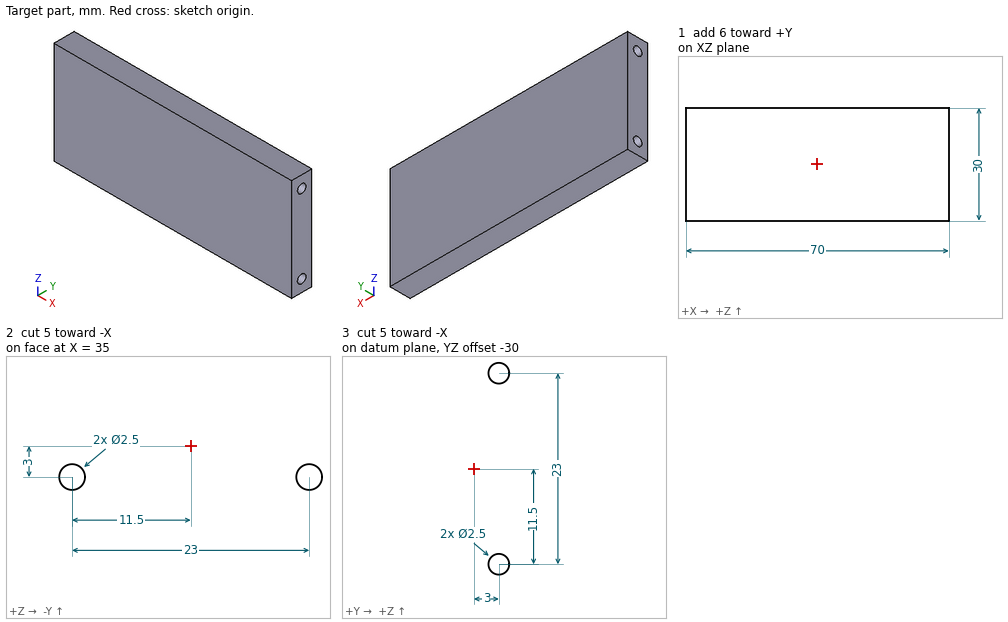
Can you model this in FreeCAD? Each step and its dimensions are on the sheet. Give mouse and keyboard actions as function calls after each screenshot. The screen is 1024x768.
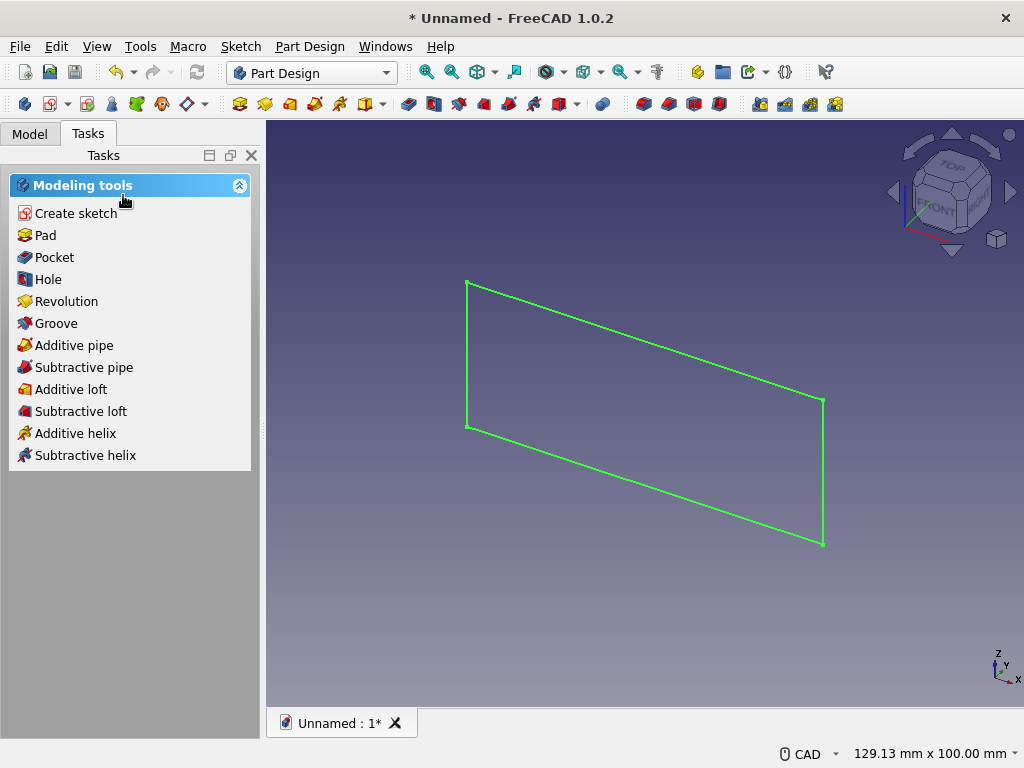
click(240, 104)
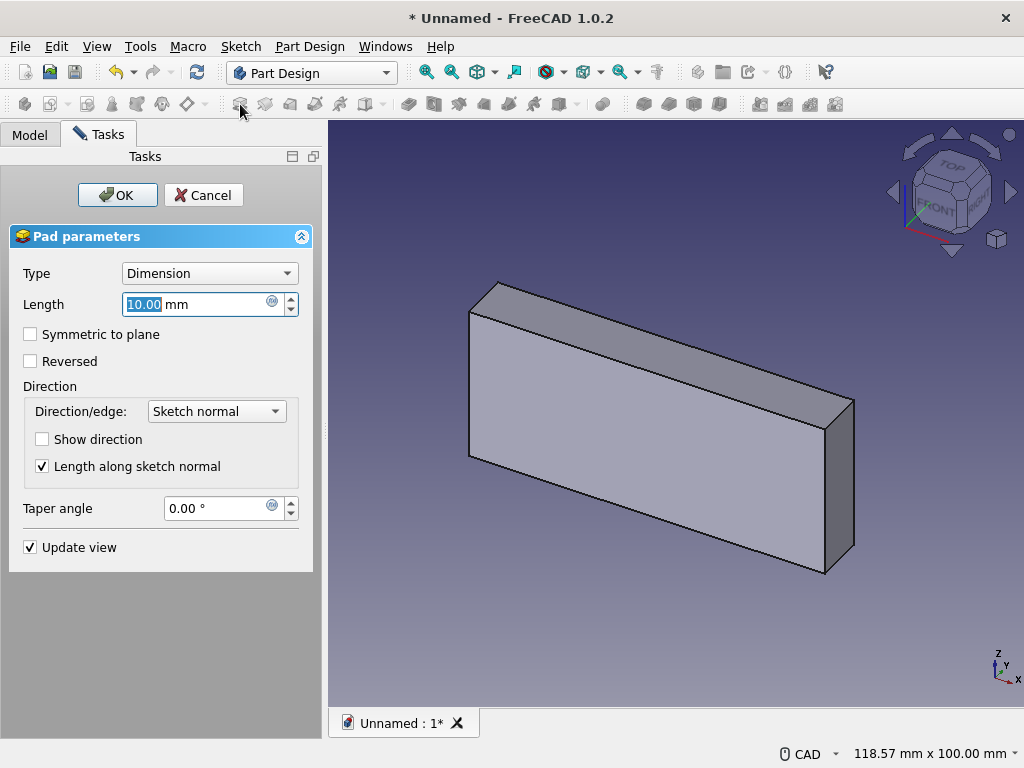
text(6)
key(Tab)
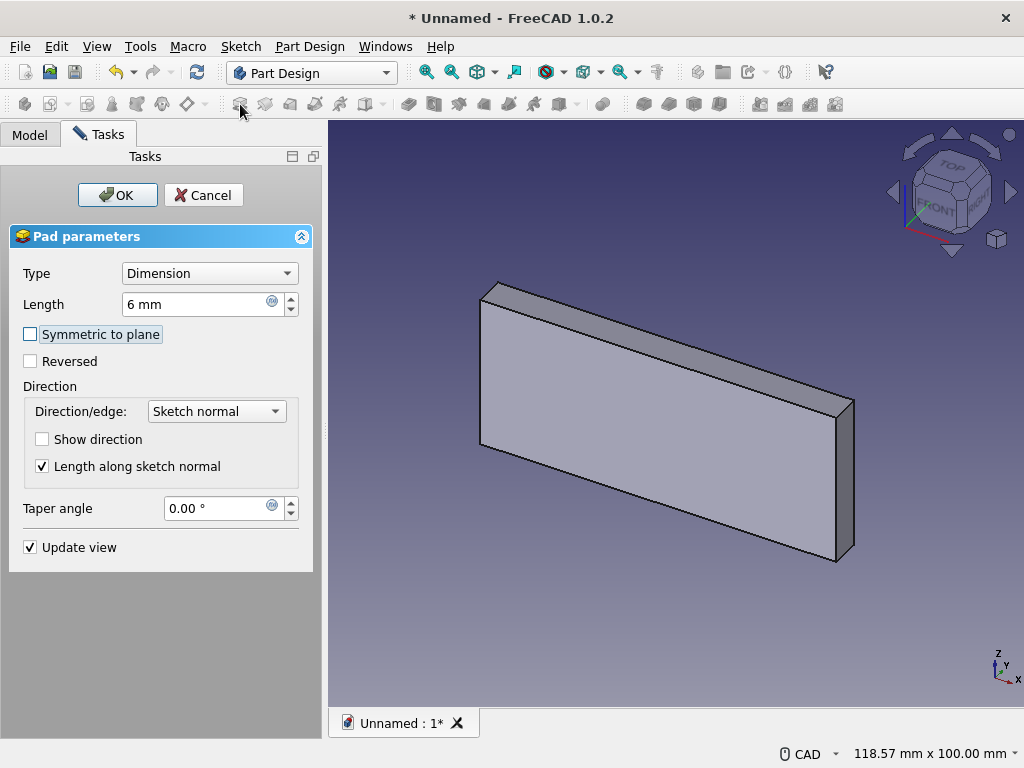
click(31, 361)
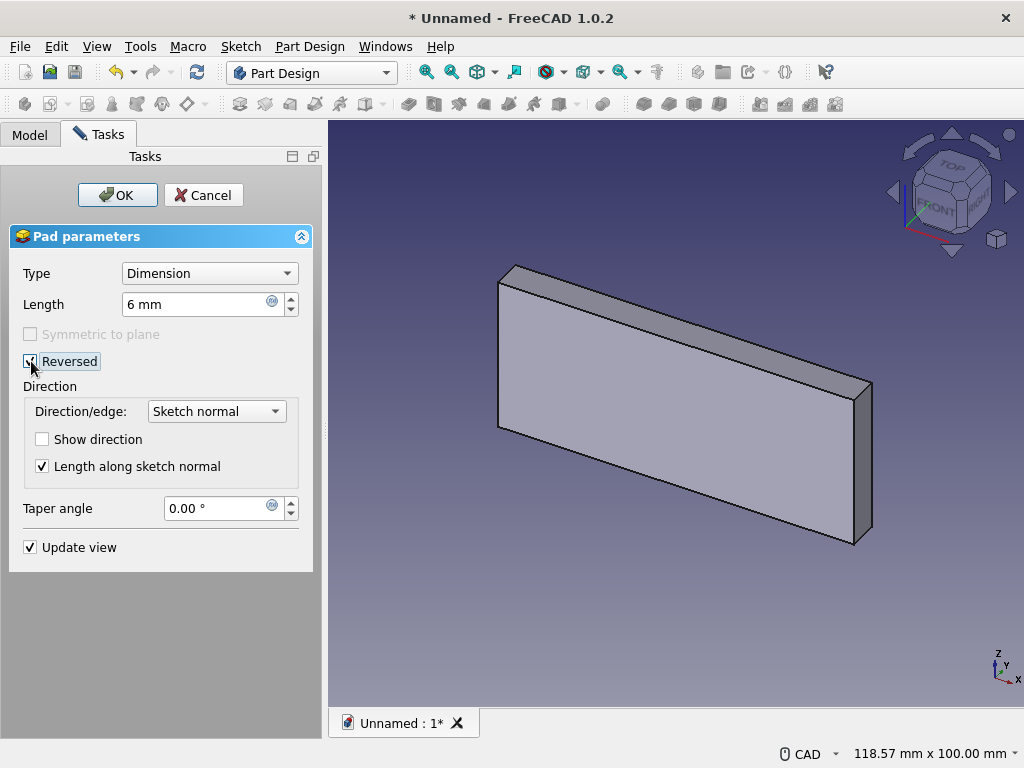
click(118, 195)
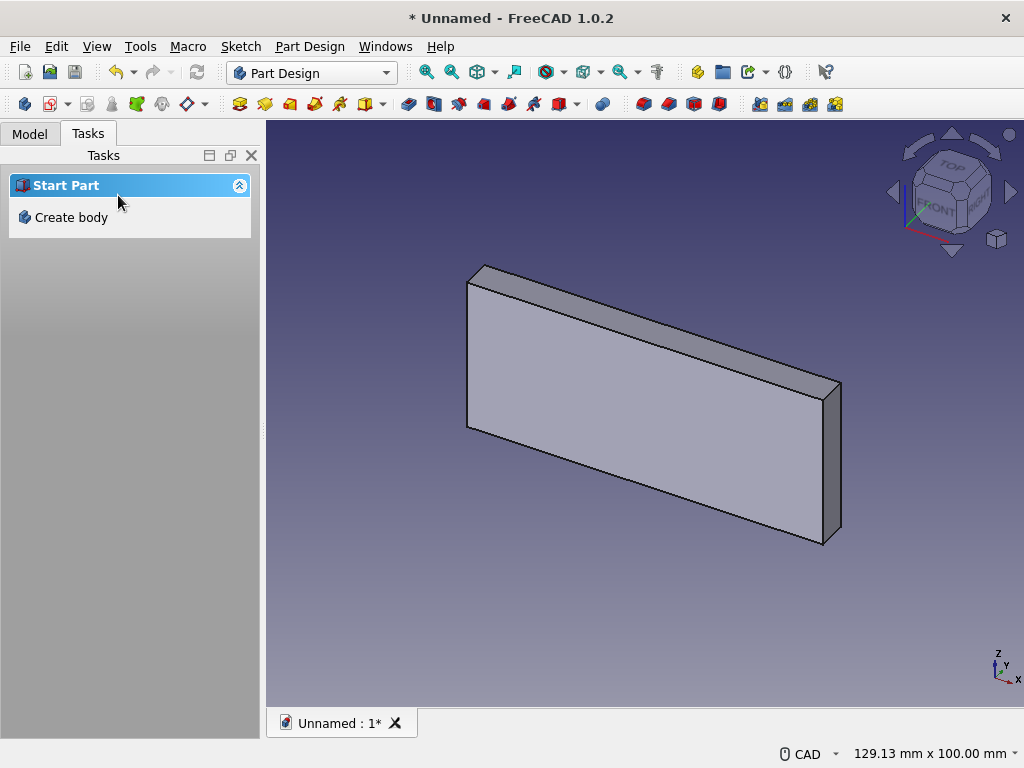
click(832, 442)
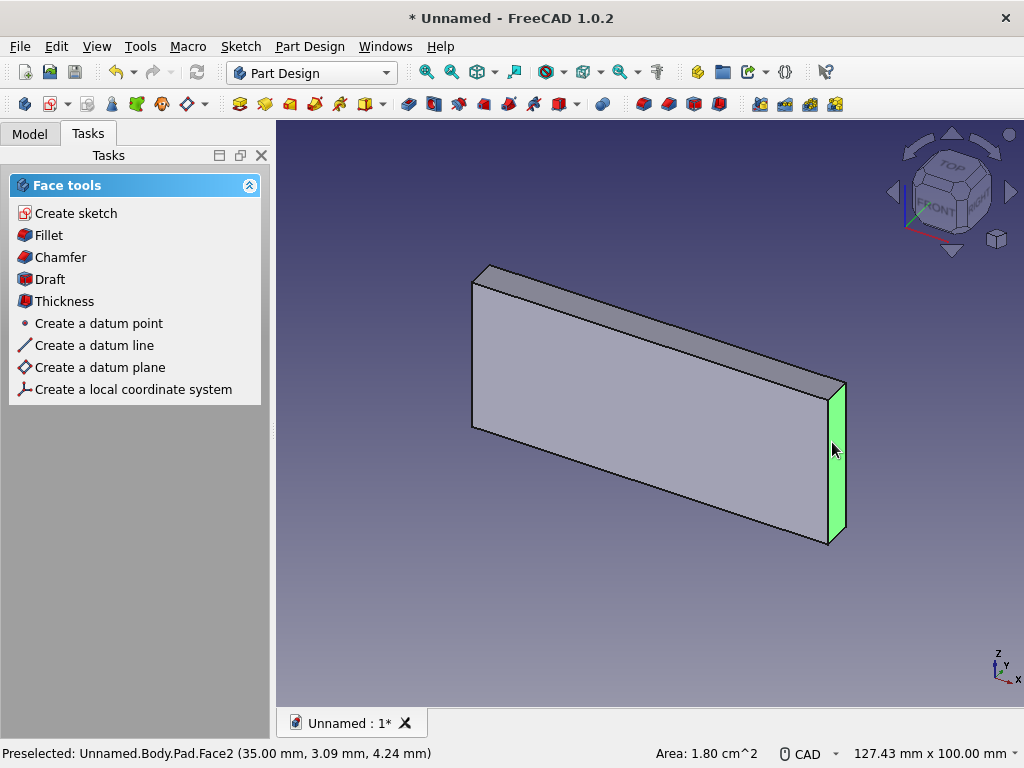
click(50, 104)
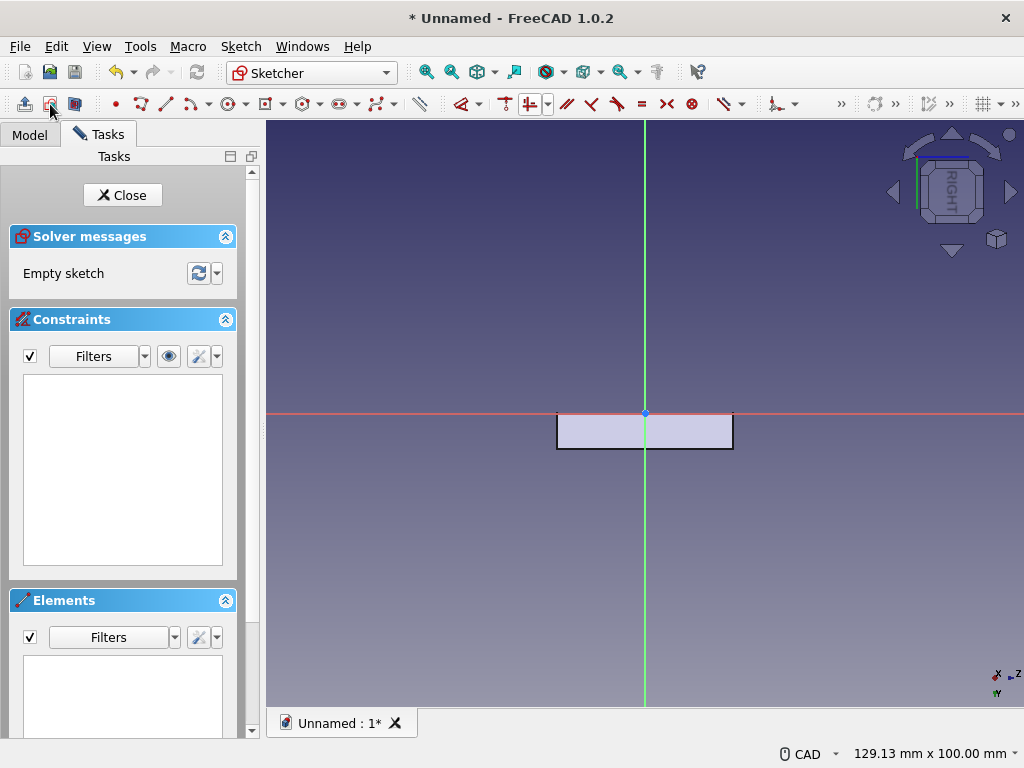
scroll(685, 433, up, 5)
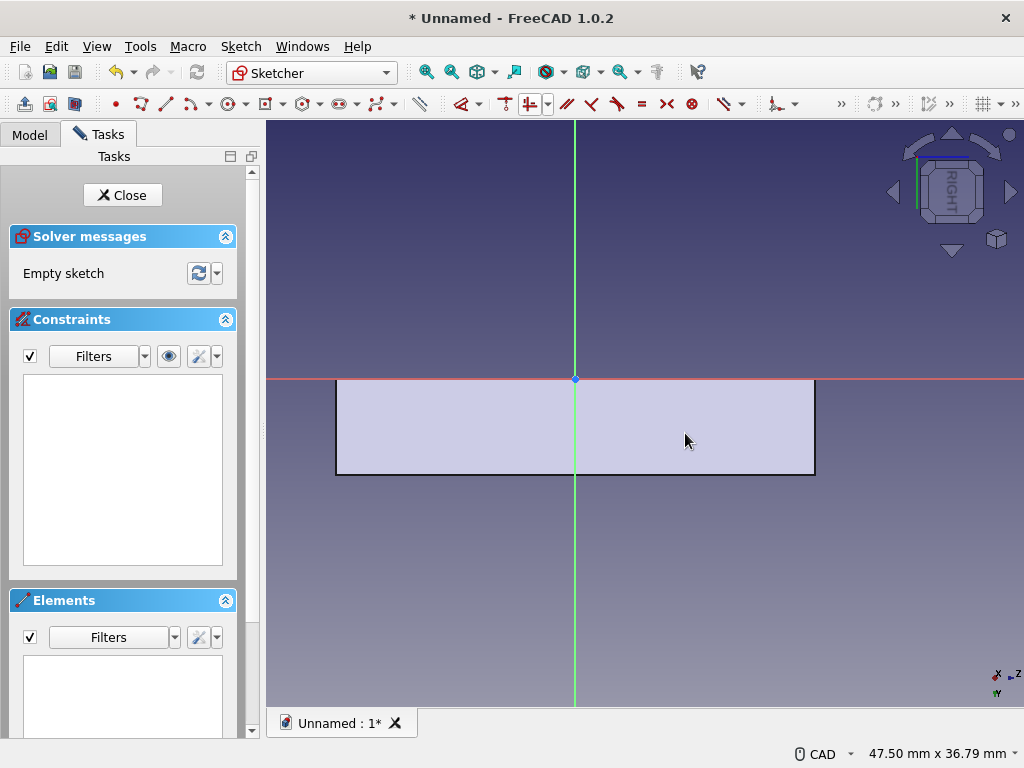
click(228, 104)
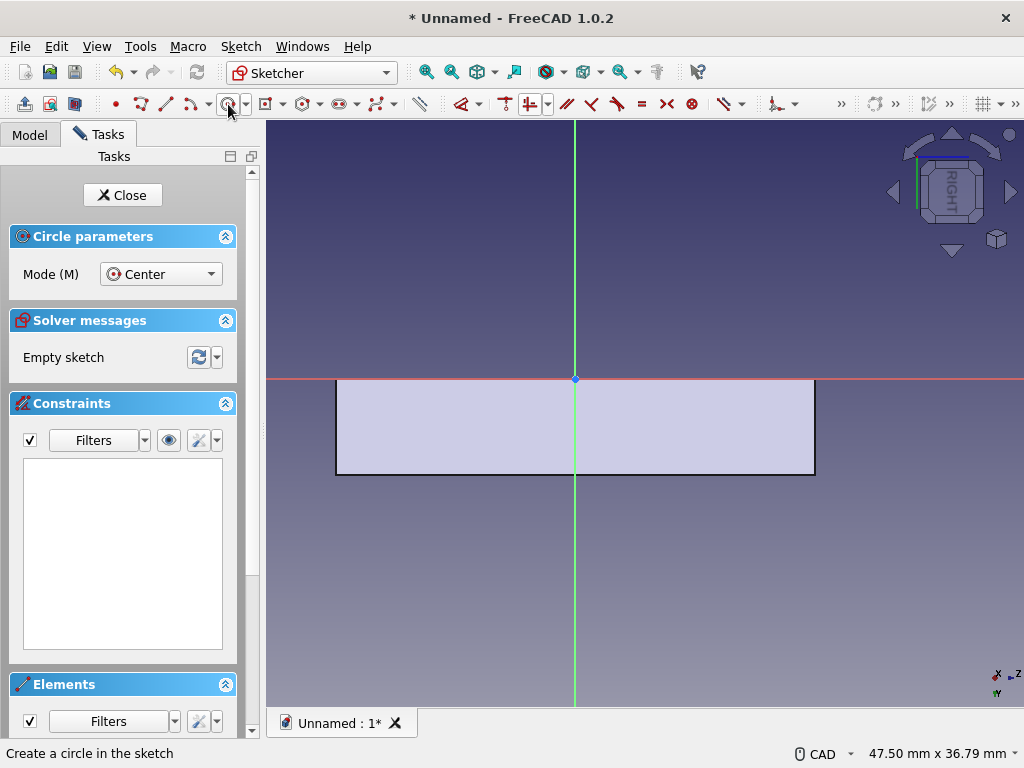
click(392, 427)
click(406, 413)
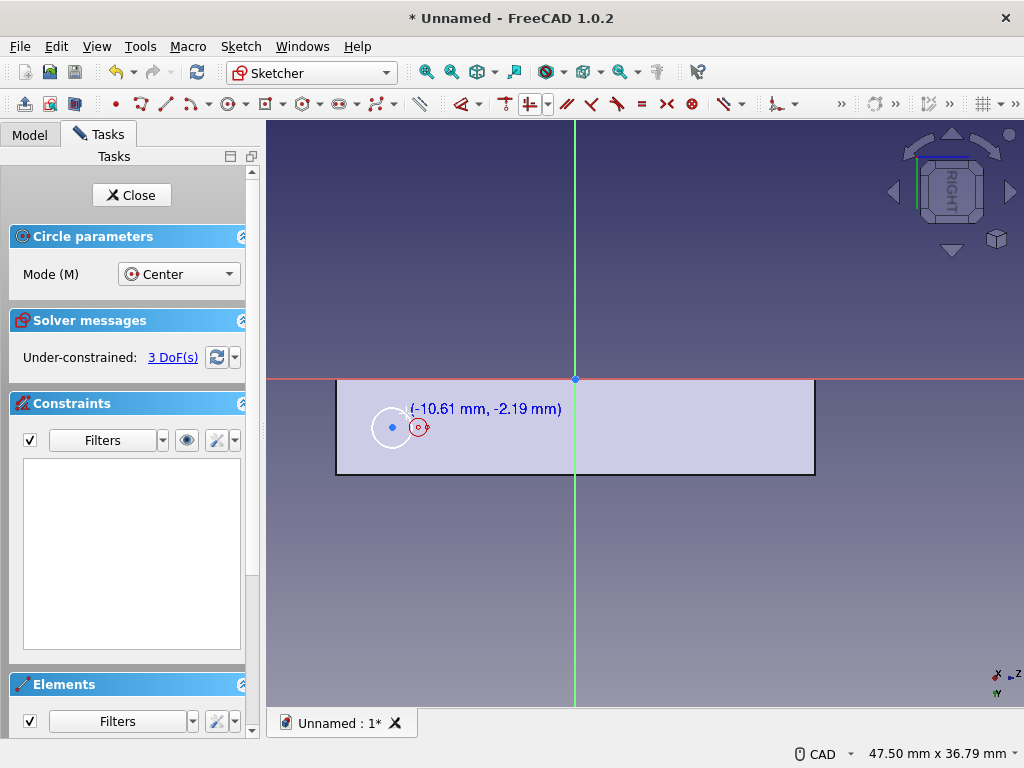
click(759, 427)
click(773, 413)
key(Escape)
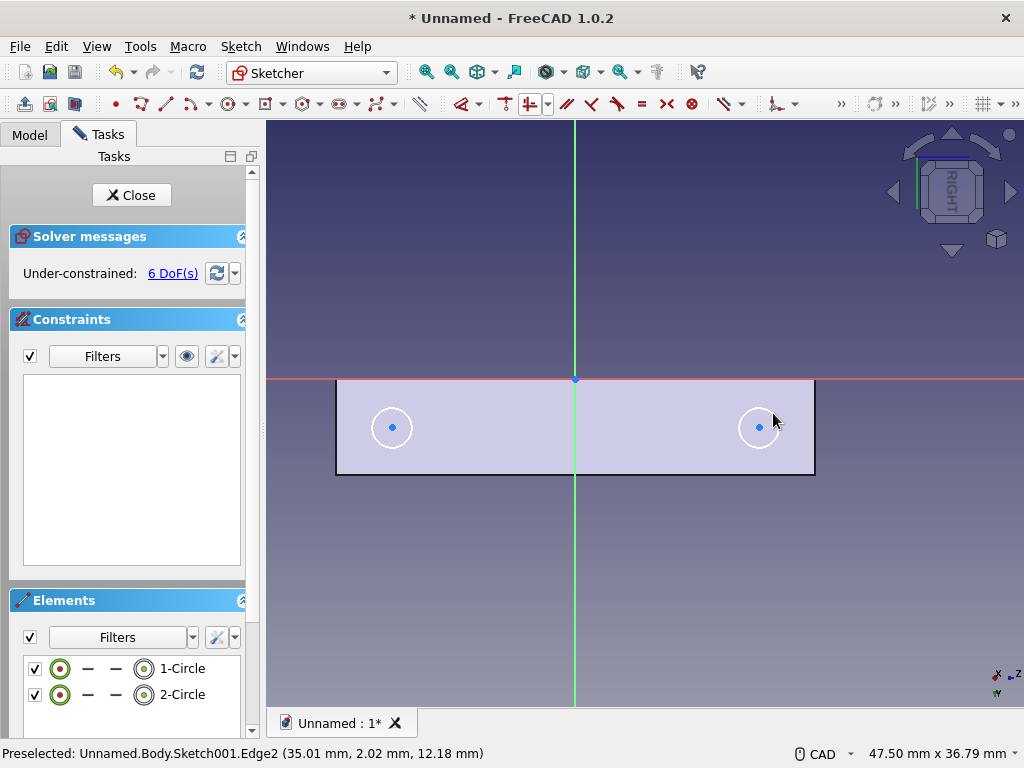
click(406, 414)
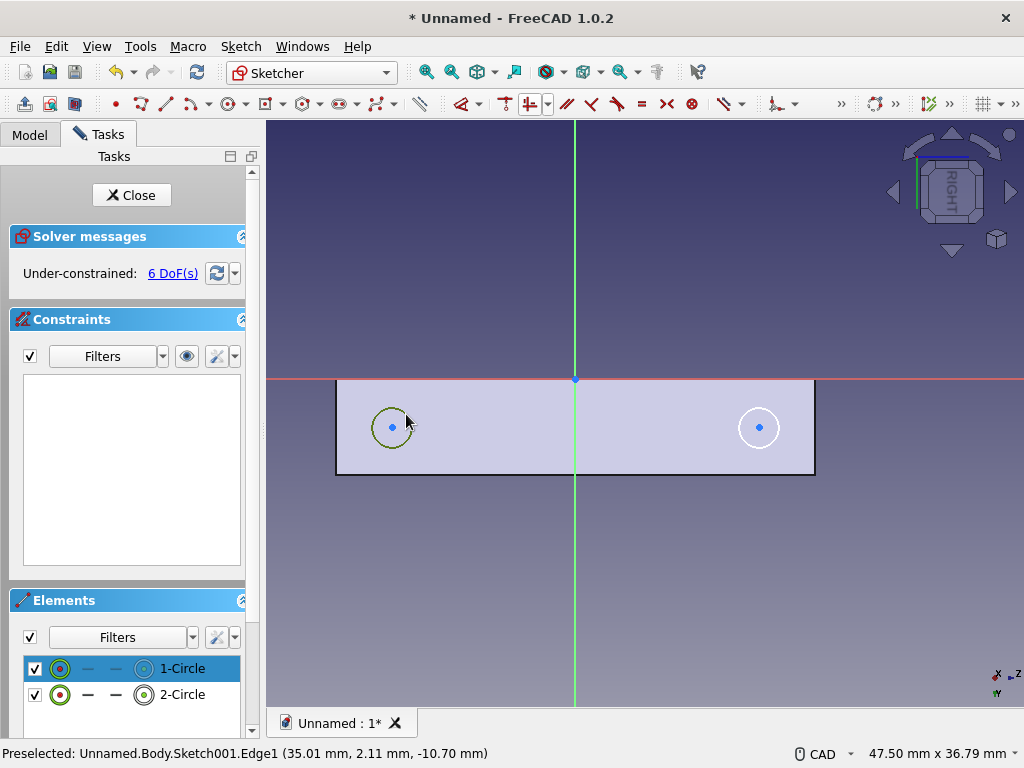
click(773, 414)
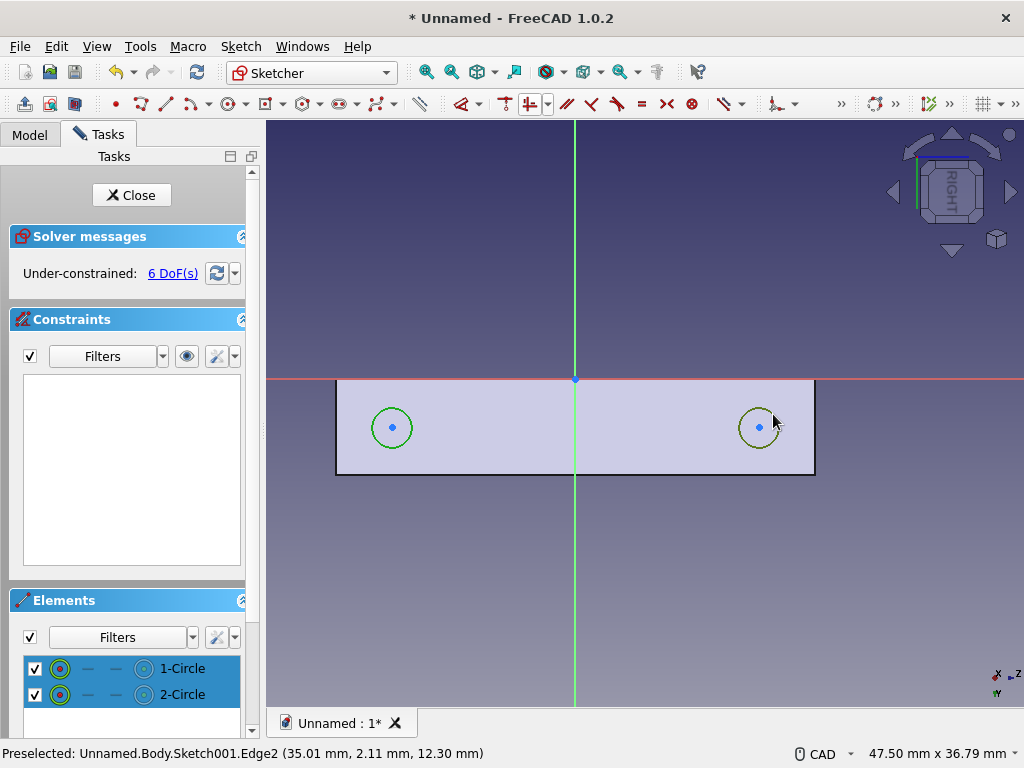
key(e)